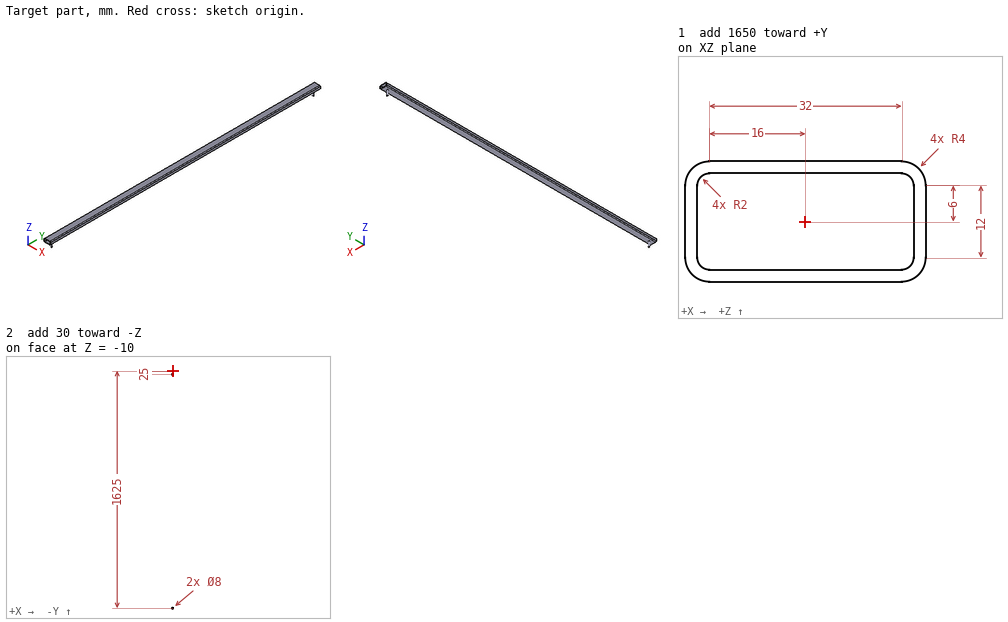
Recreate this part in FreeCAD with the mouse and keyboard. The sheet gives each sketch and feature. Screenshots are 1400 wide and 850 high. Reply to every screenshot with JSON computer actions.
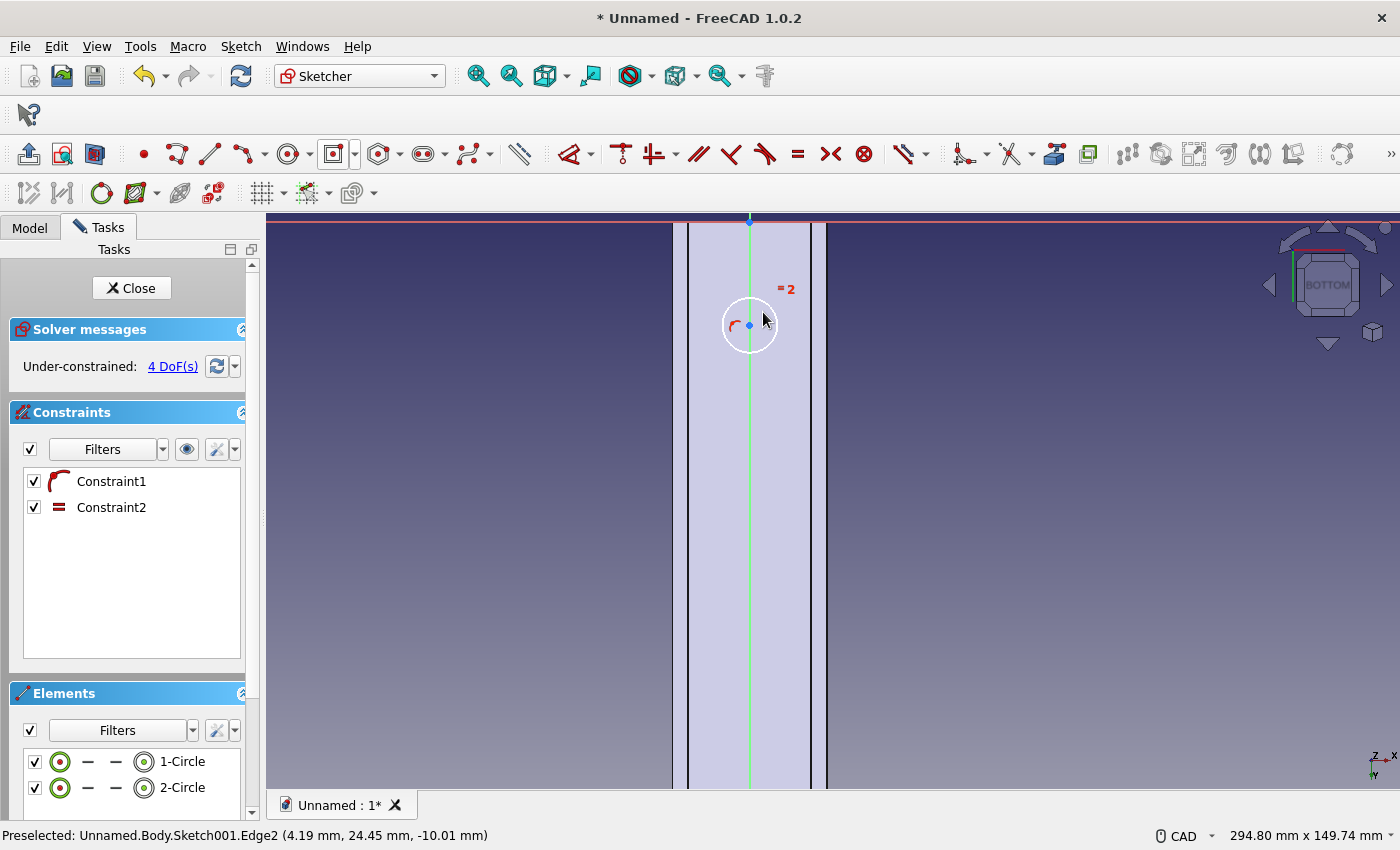
{"action": "scroll", "coordinate": [765, 316], "scroll_direction": "down", "scroll_amount": 14}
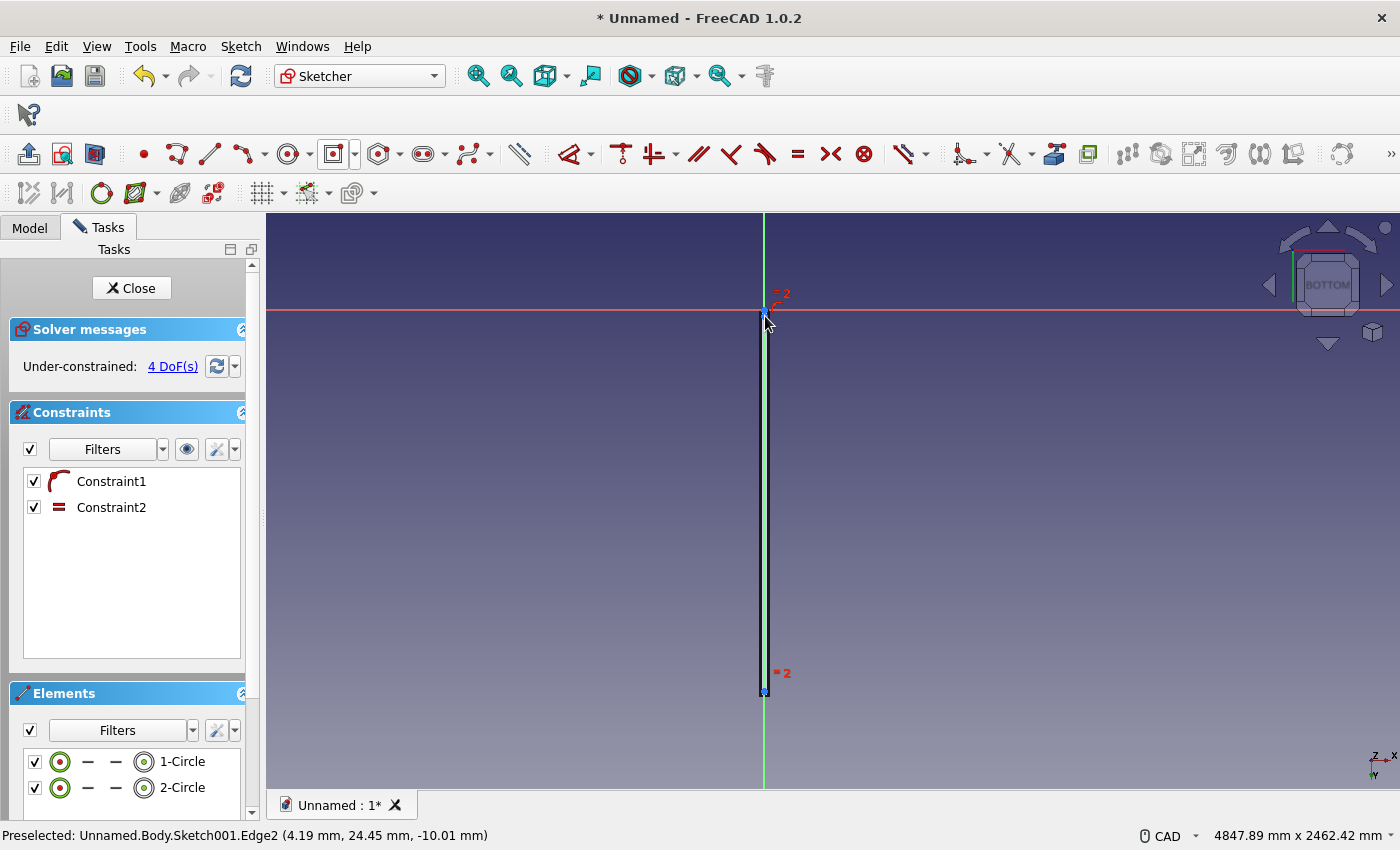
{"action": "left_click", "coordinate": [764, 691]}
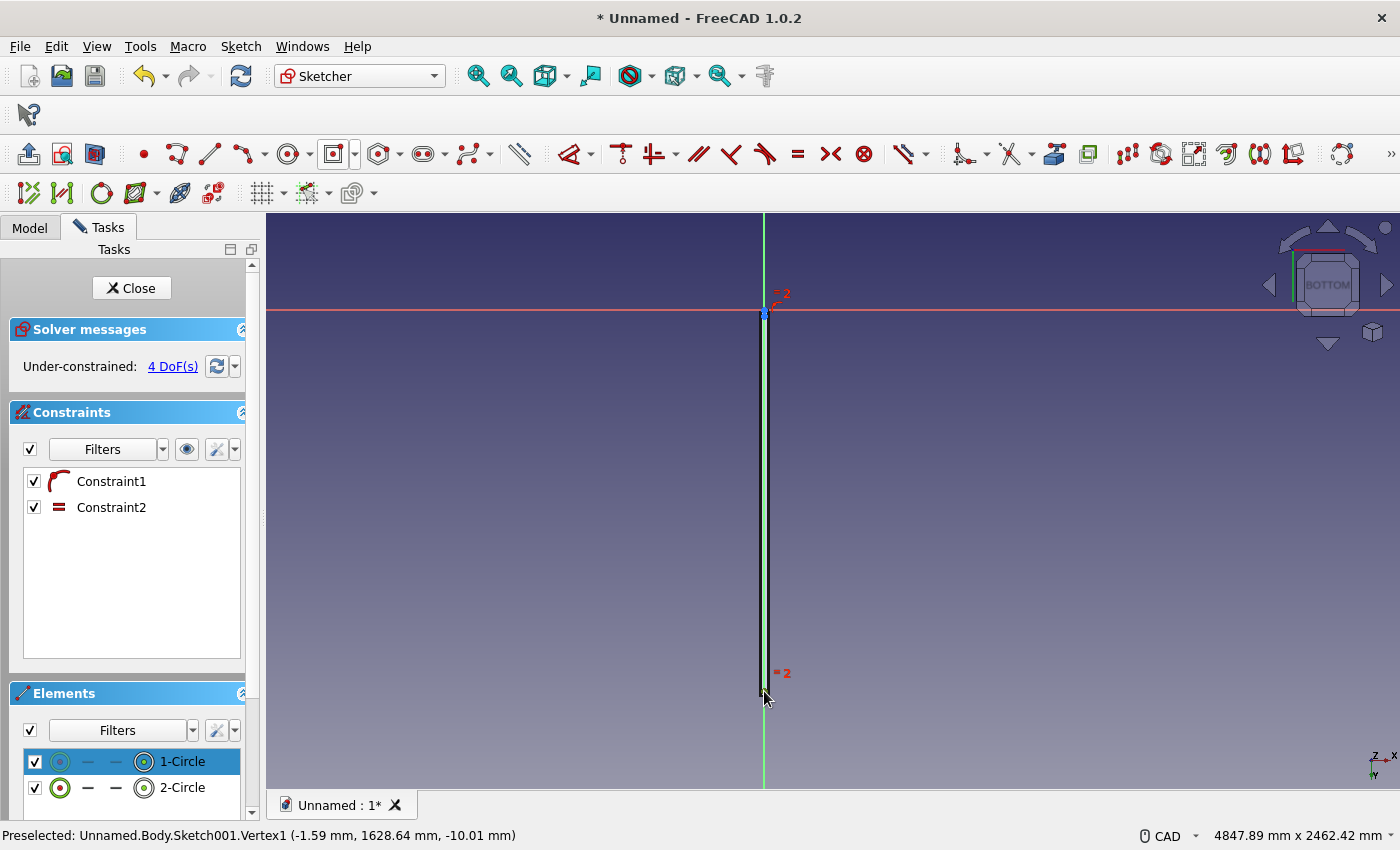
{"action": "left_click", "coordinate": [764, 724]}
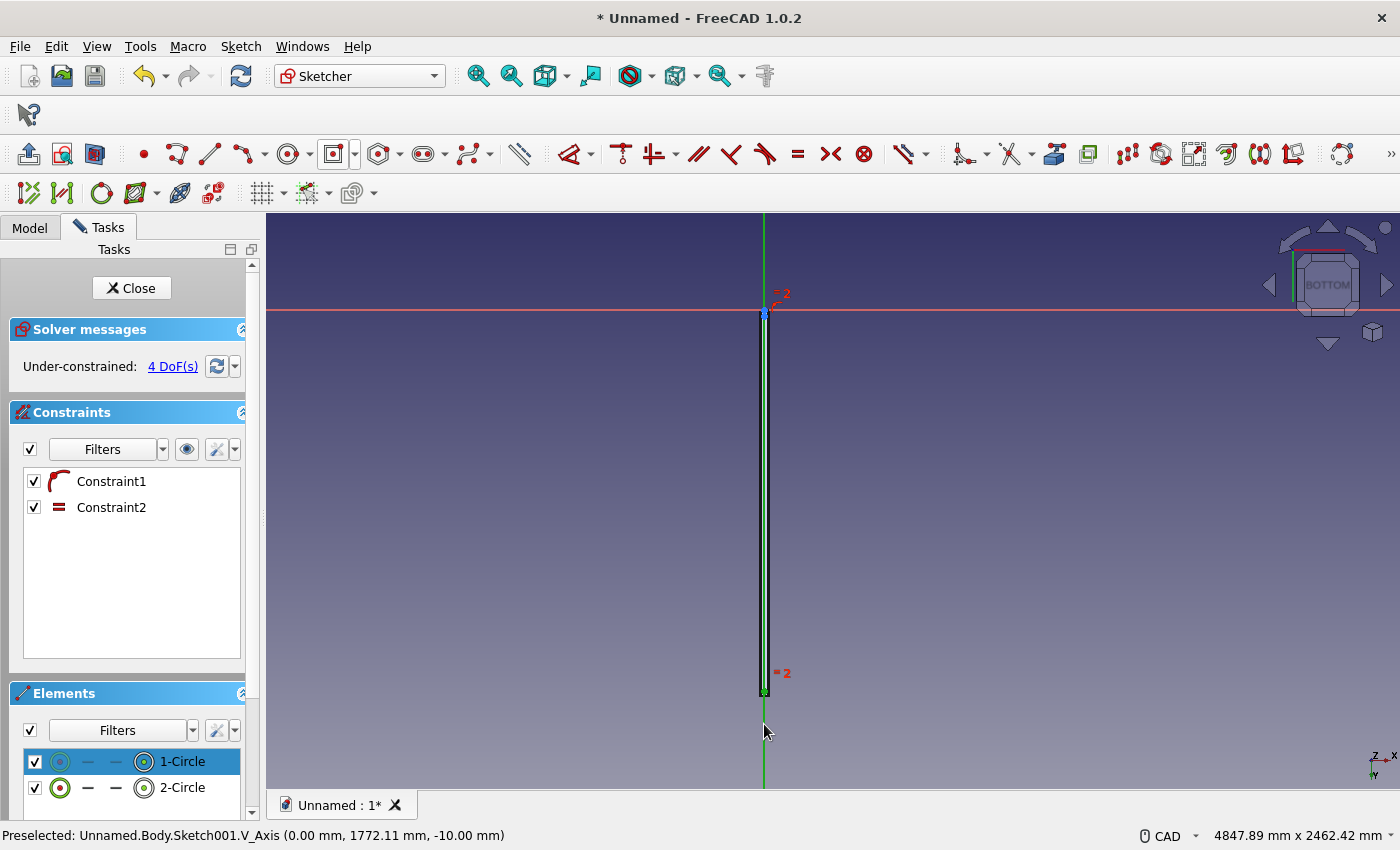
{"action": "left_click", "coordinate": [621, 154]}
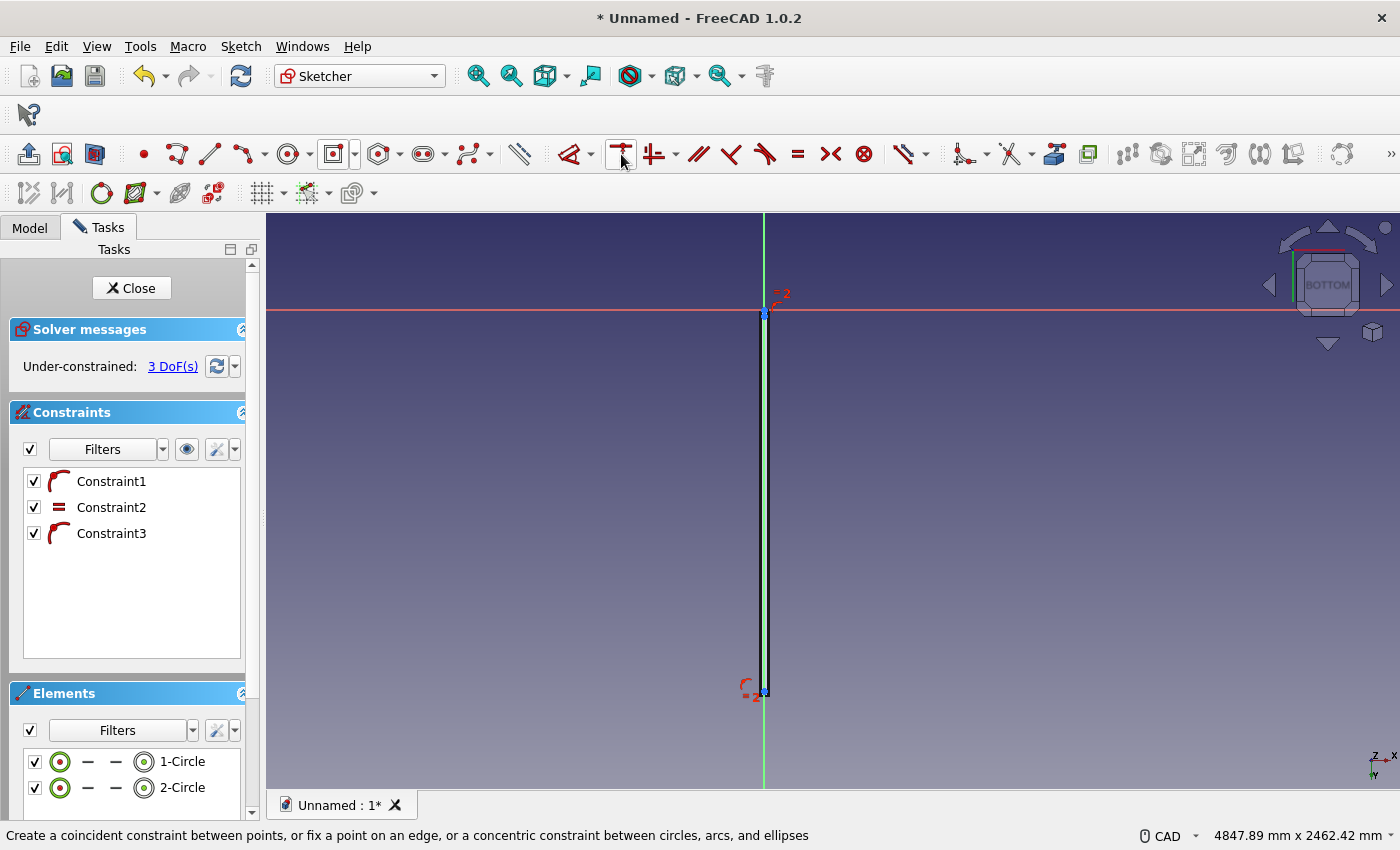
{"action": "key", "text": "d"}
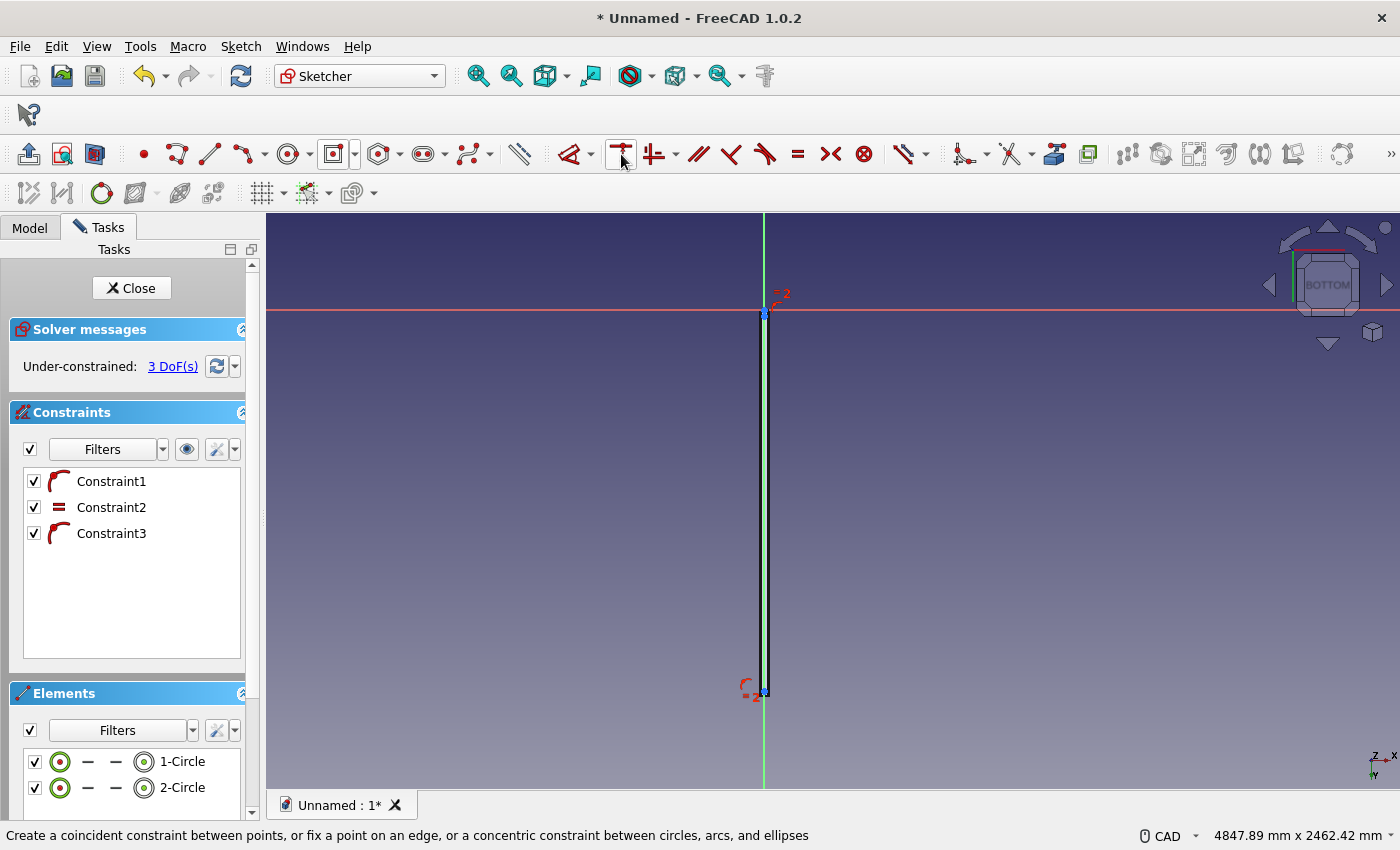
{"action": "scroll", "coordinate": [765, 690], "scroll_direction": "up", "scroll_amount": 16}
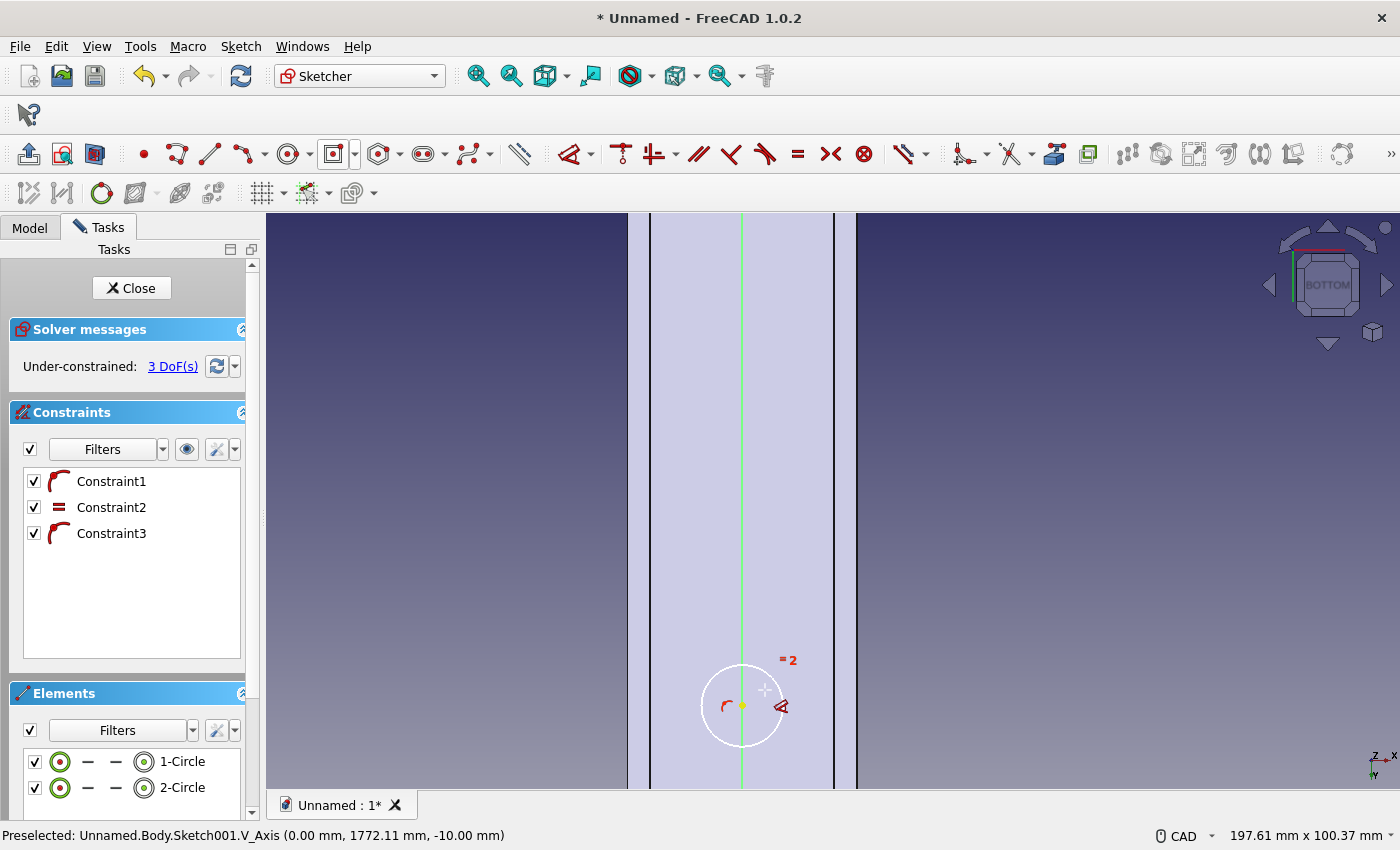
{"action": "left_click", "coordinate": [743, 665]}
{"action": "left_click", "coordinate": [778, 643]}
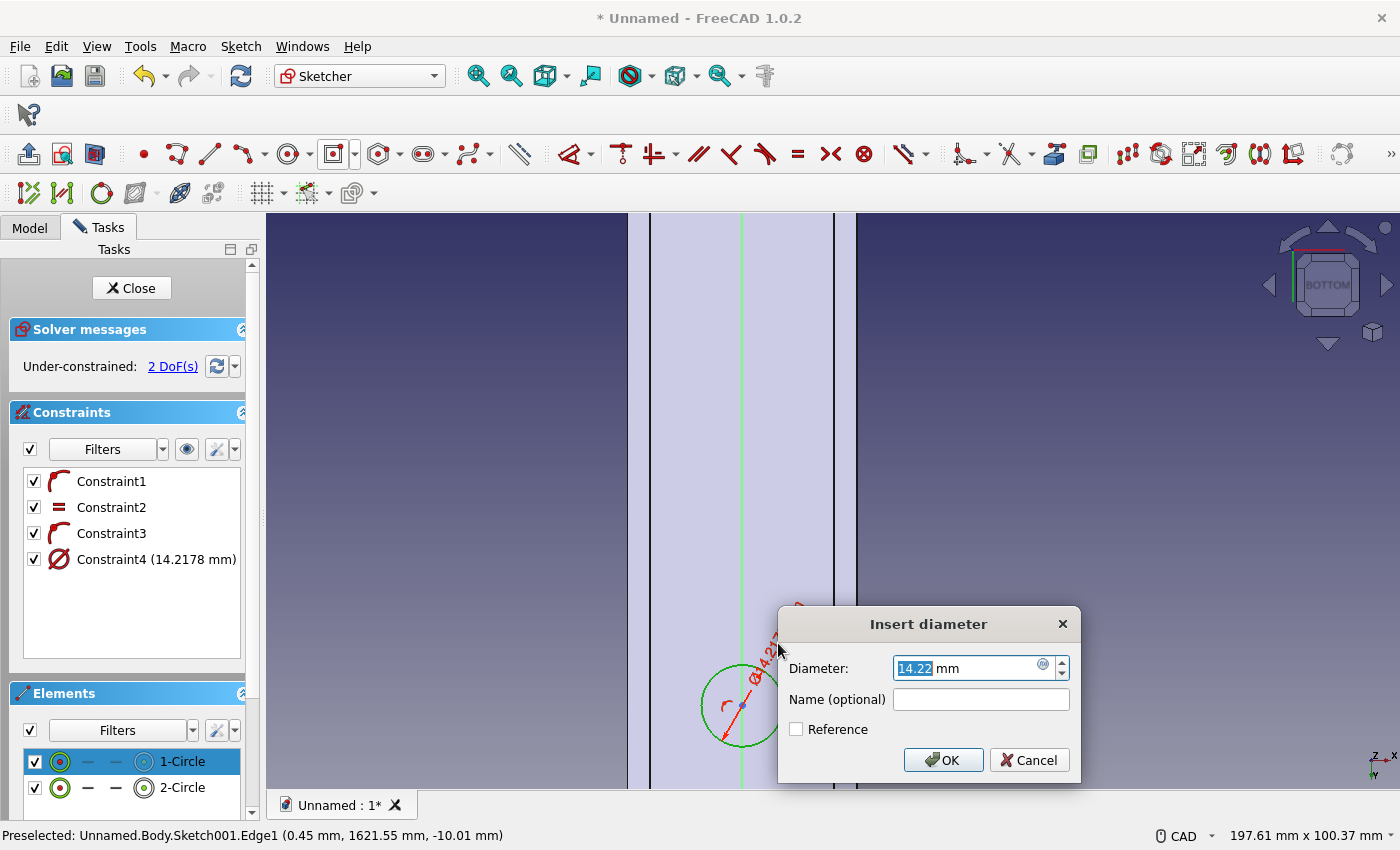
{"action": "type", "text": "8"}
{"action": "key", "text": "Return"}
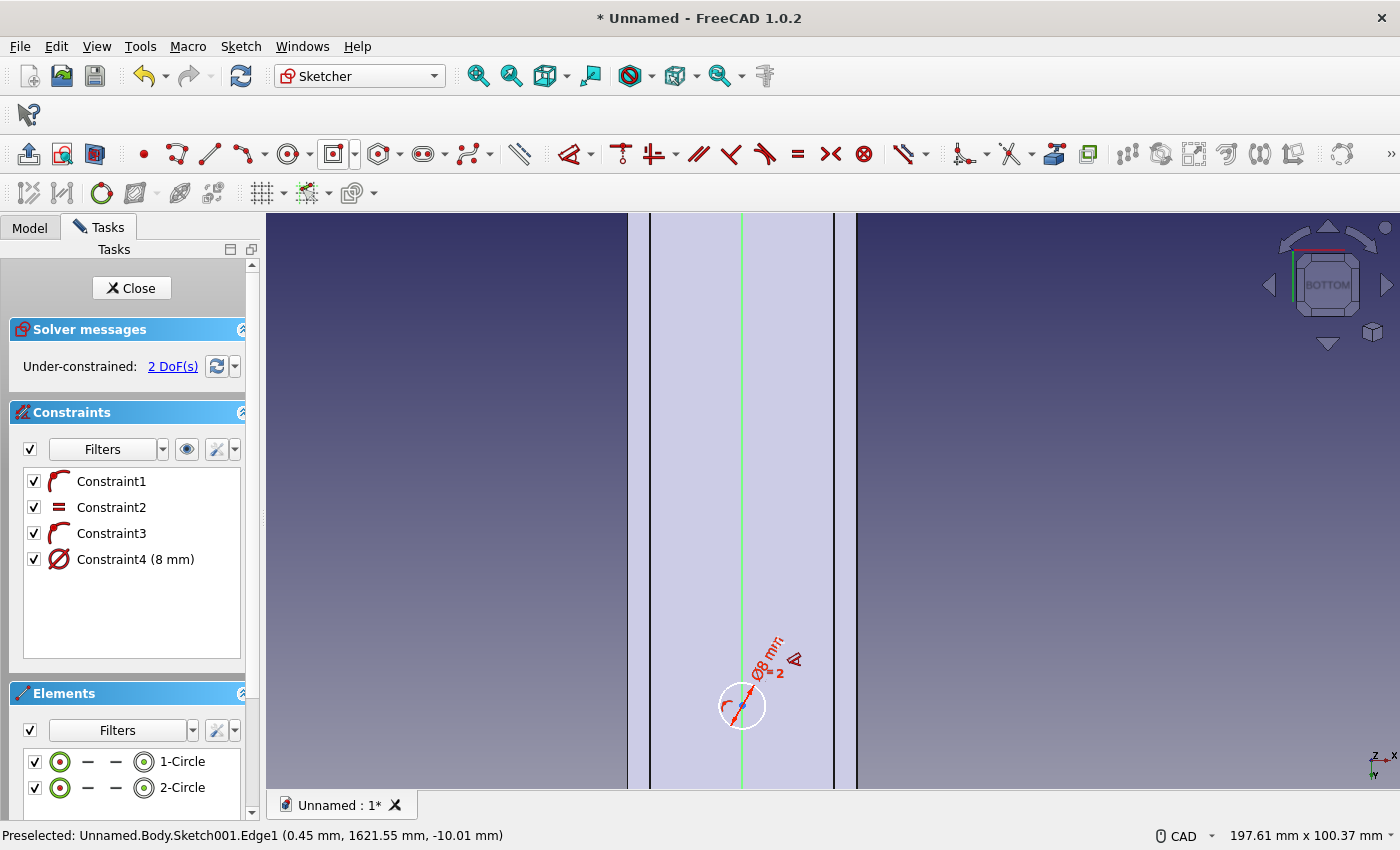
{"action": "scroll", "coordinate": [766, 735], "scroll_direction": "down", "scroll_amount": 15}